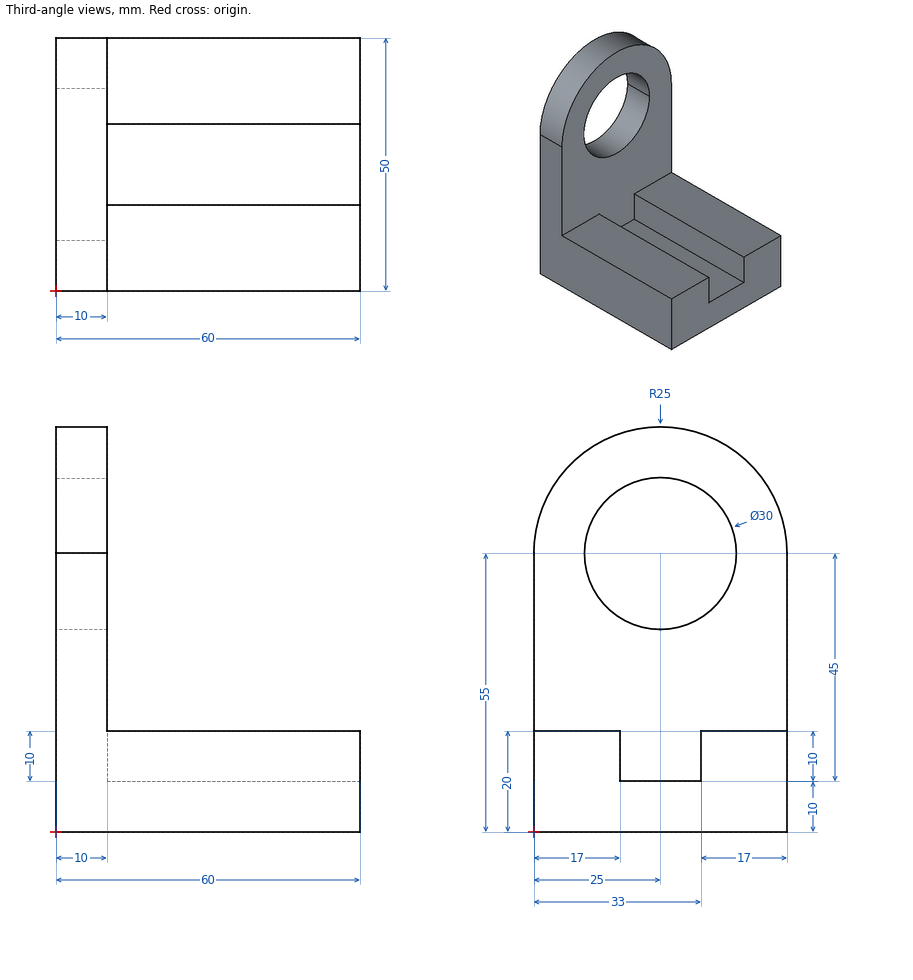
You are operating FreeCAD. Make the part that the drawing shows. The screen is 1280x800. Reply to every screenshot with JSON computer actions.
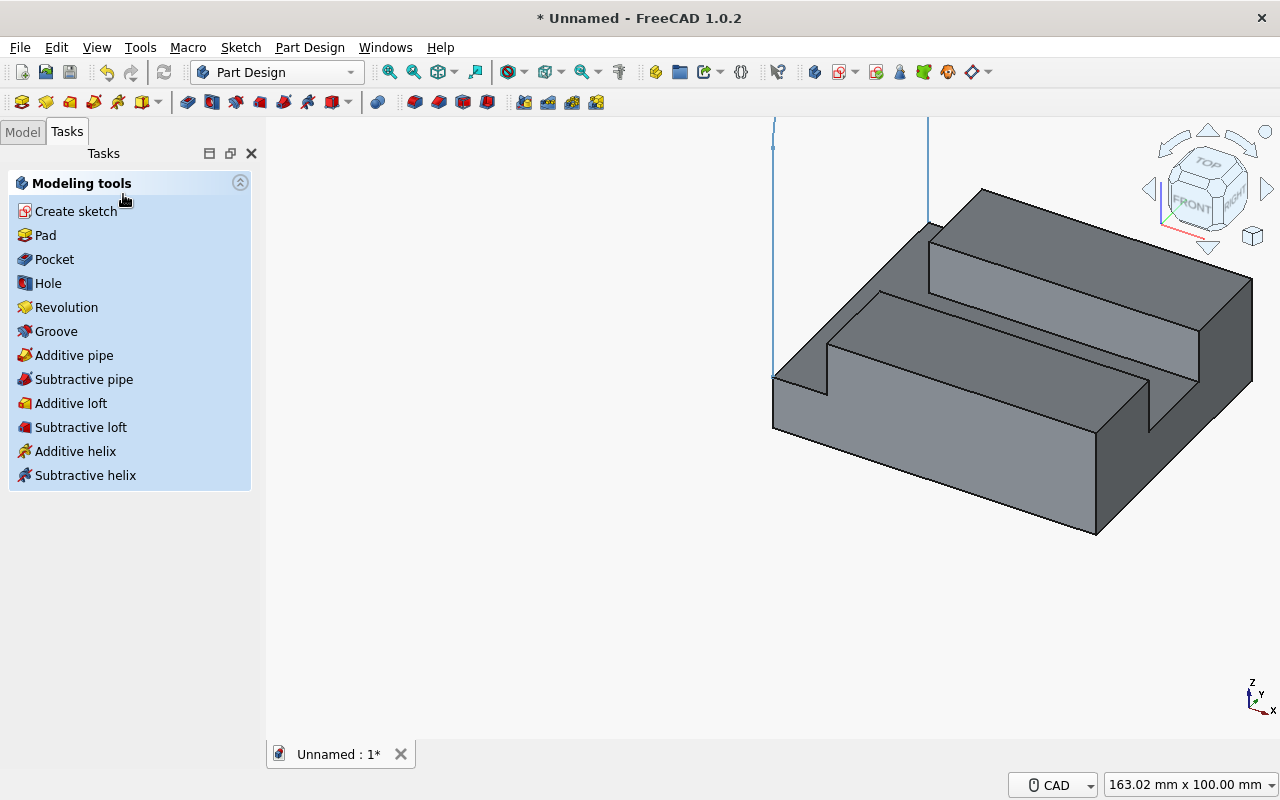
{"action": "left_click", "coordinate": [22, 102]}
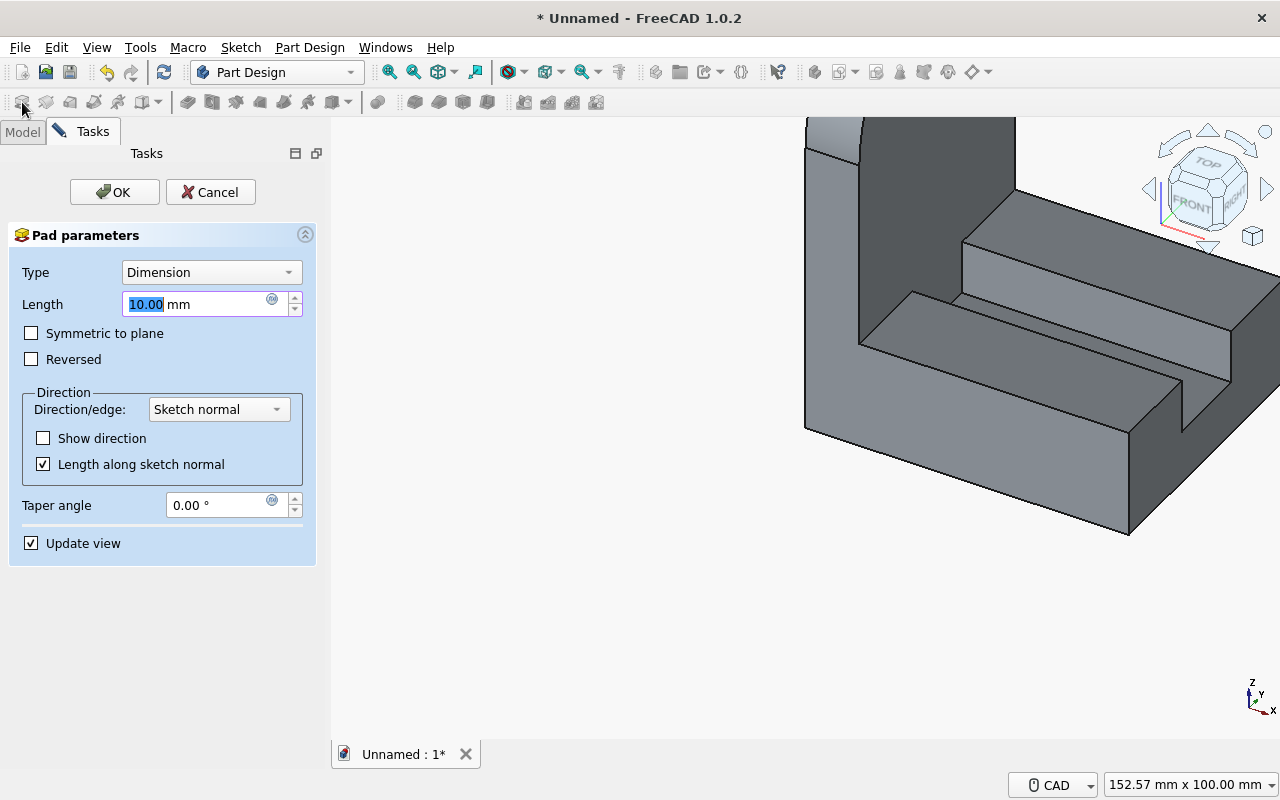
{"action": "type", "text": "10"}
{"action": "key", "text": "Tab"}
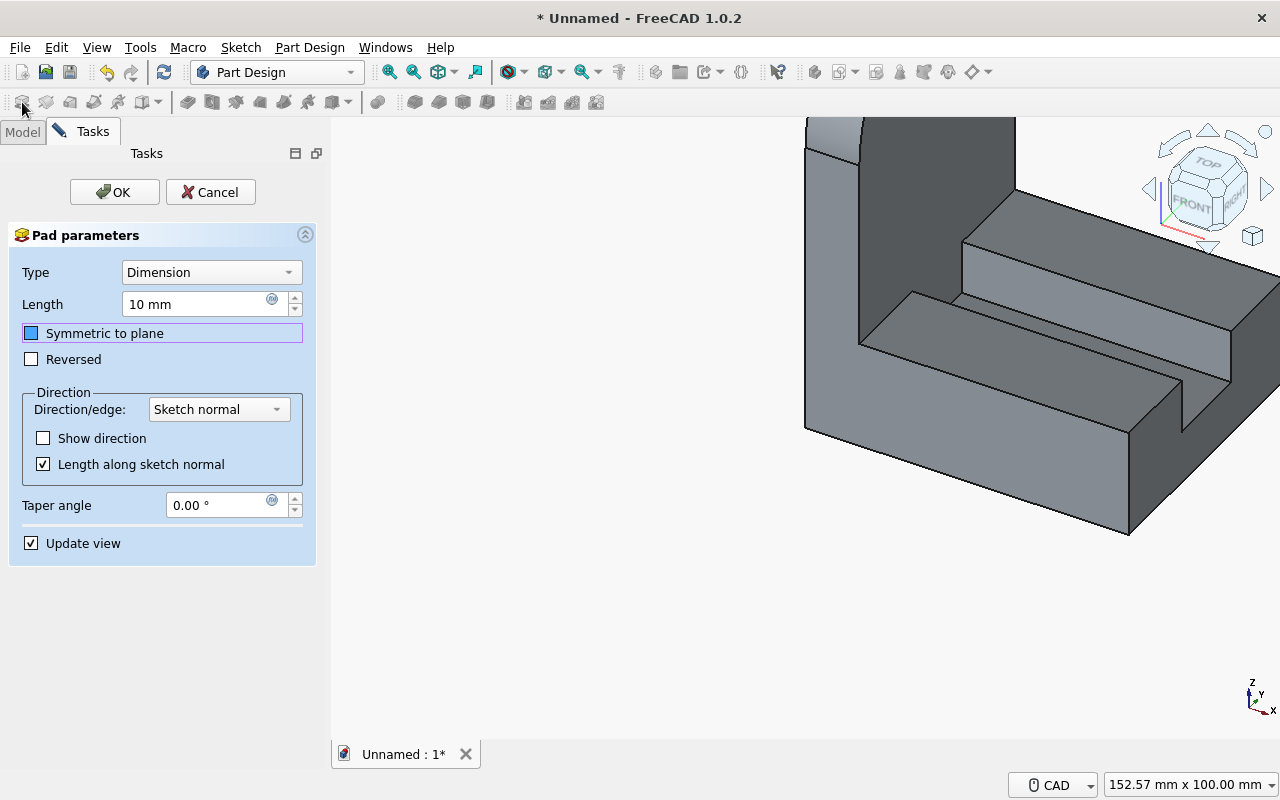
{"action": "left_click", "coordinate": [115, 192]}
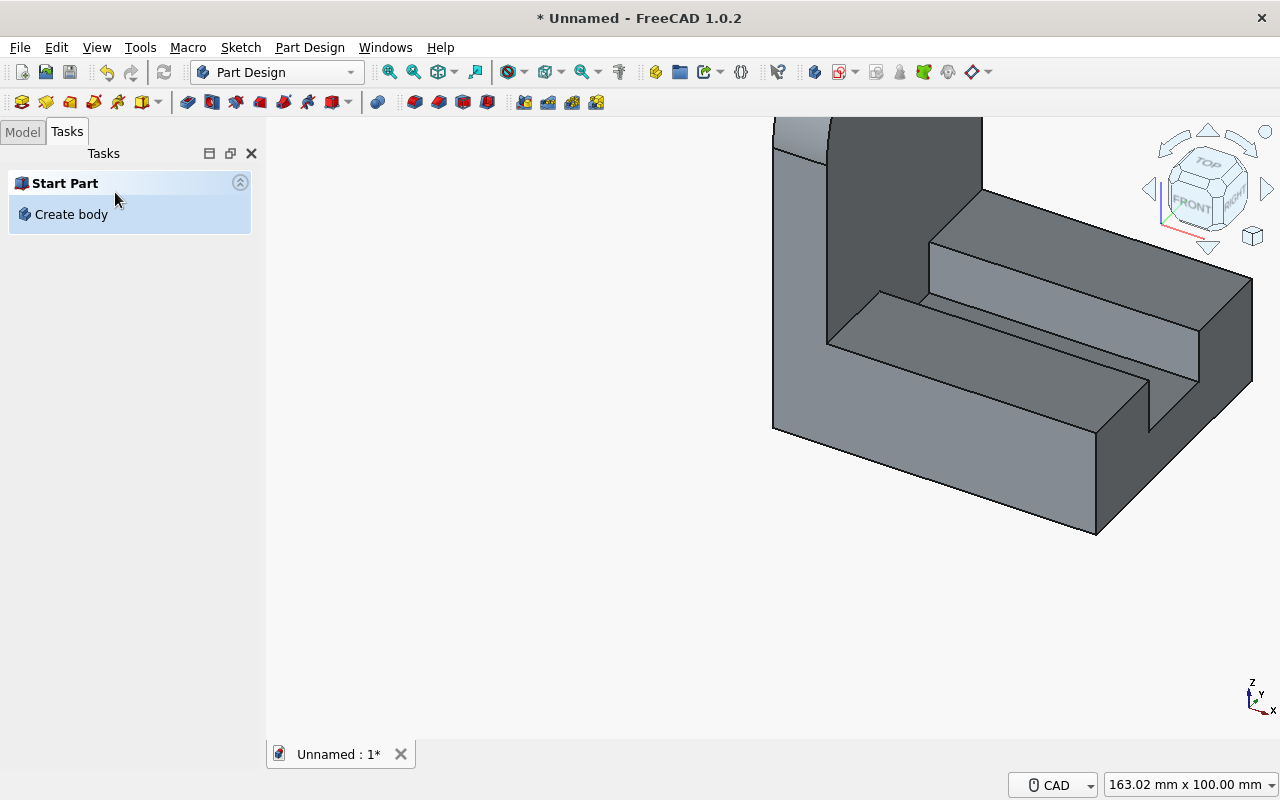
{"action": "left_click", "coordinate": [390, 72]}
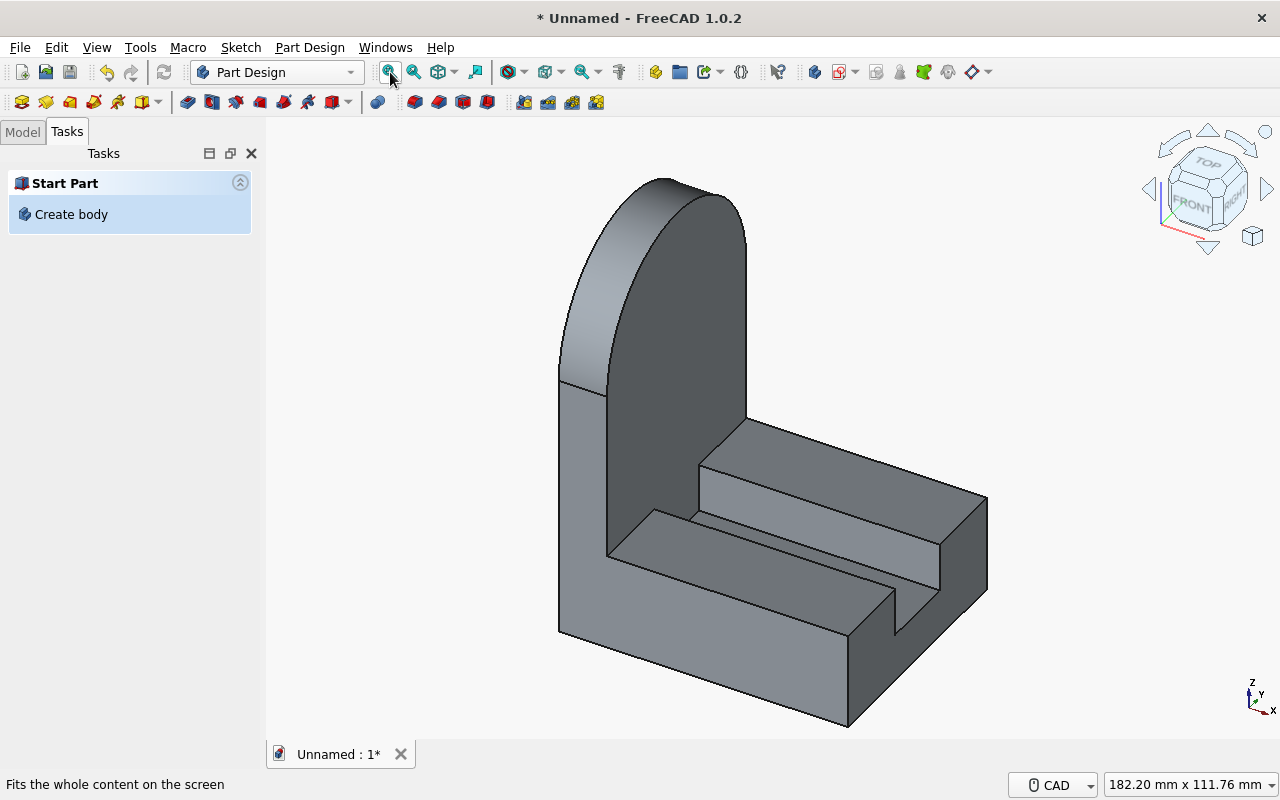
{"action": "left_click", "coordinate": [677, 327]}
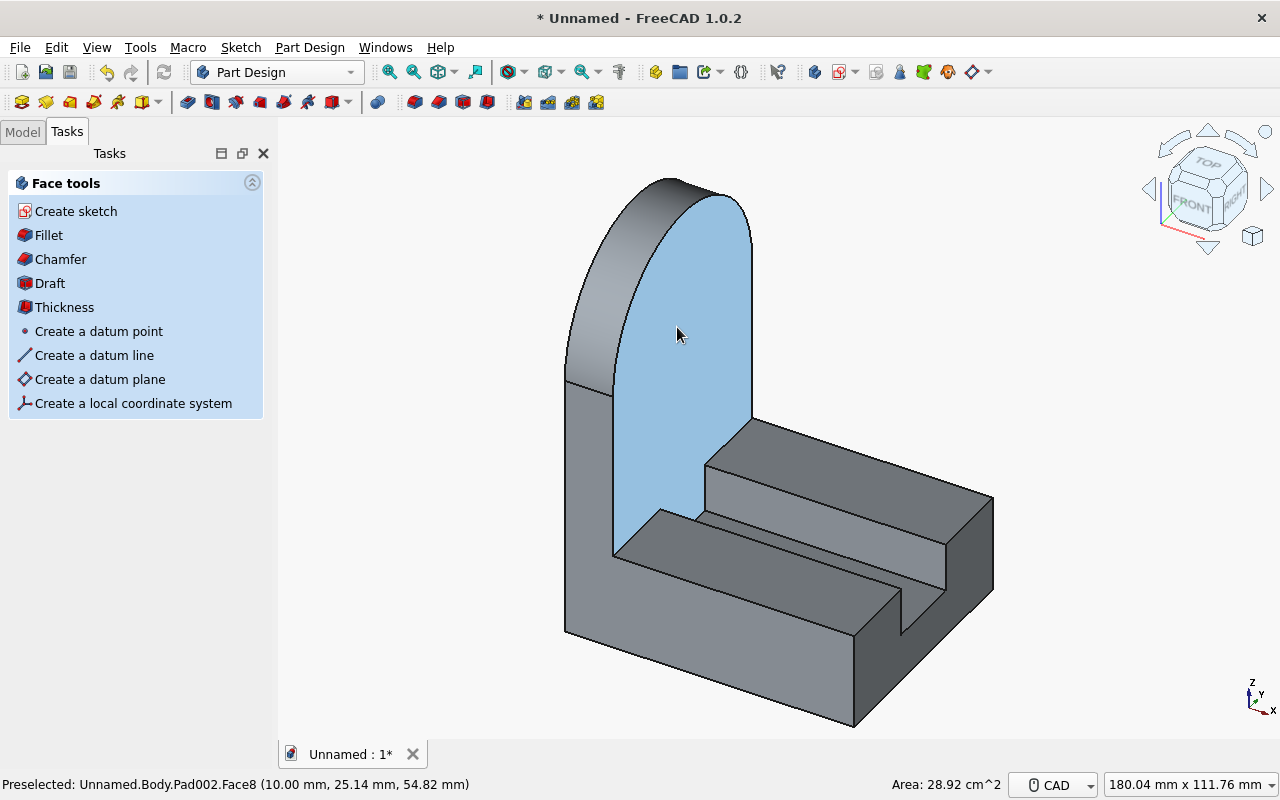
{"action": "left_click", "coordinate": [840, 72]}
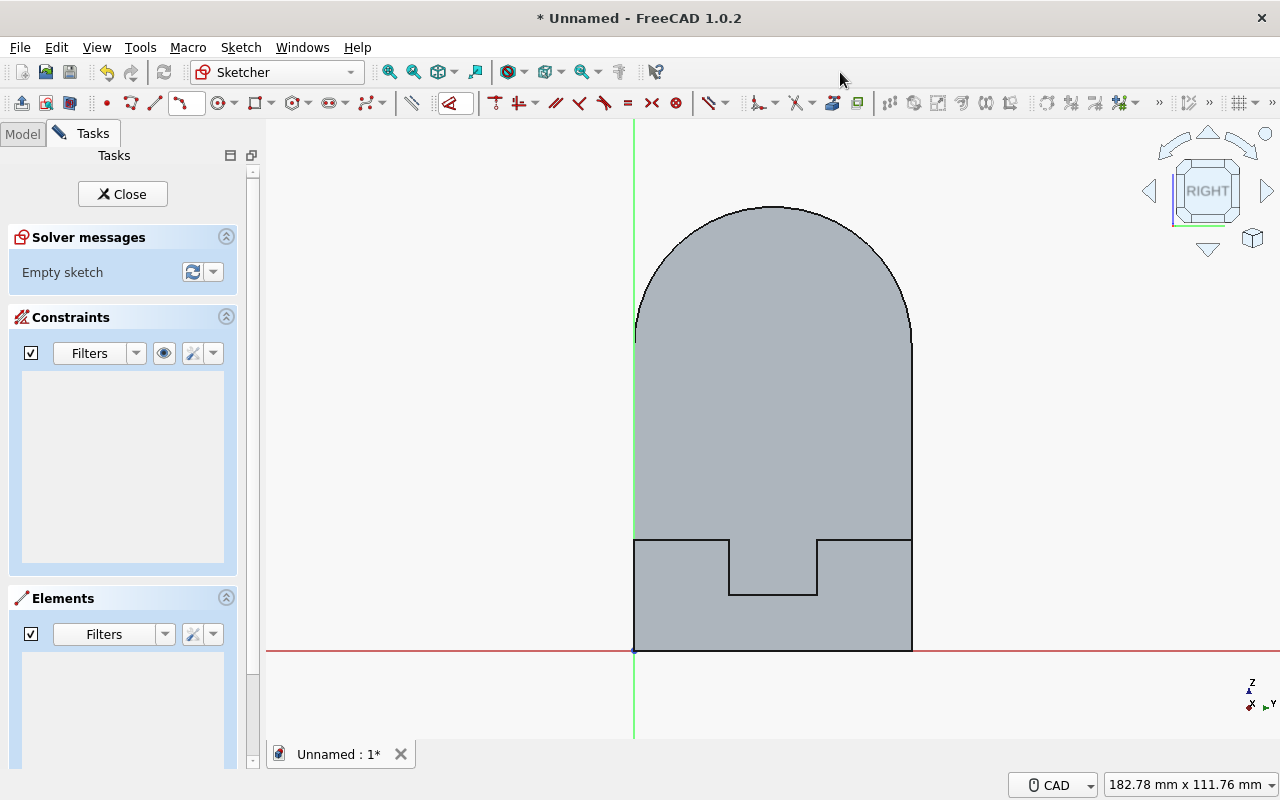
{"action": "left_click", "coordinate": [70, 104]}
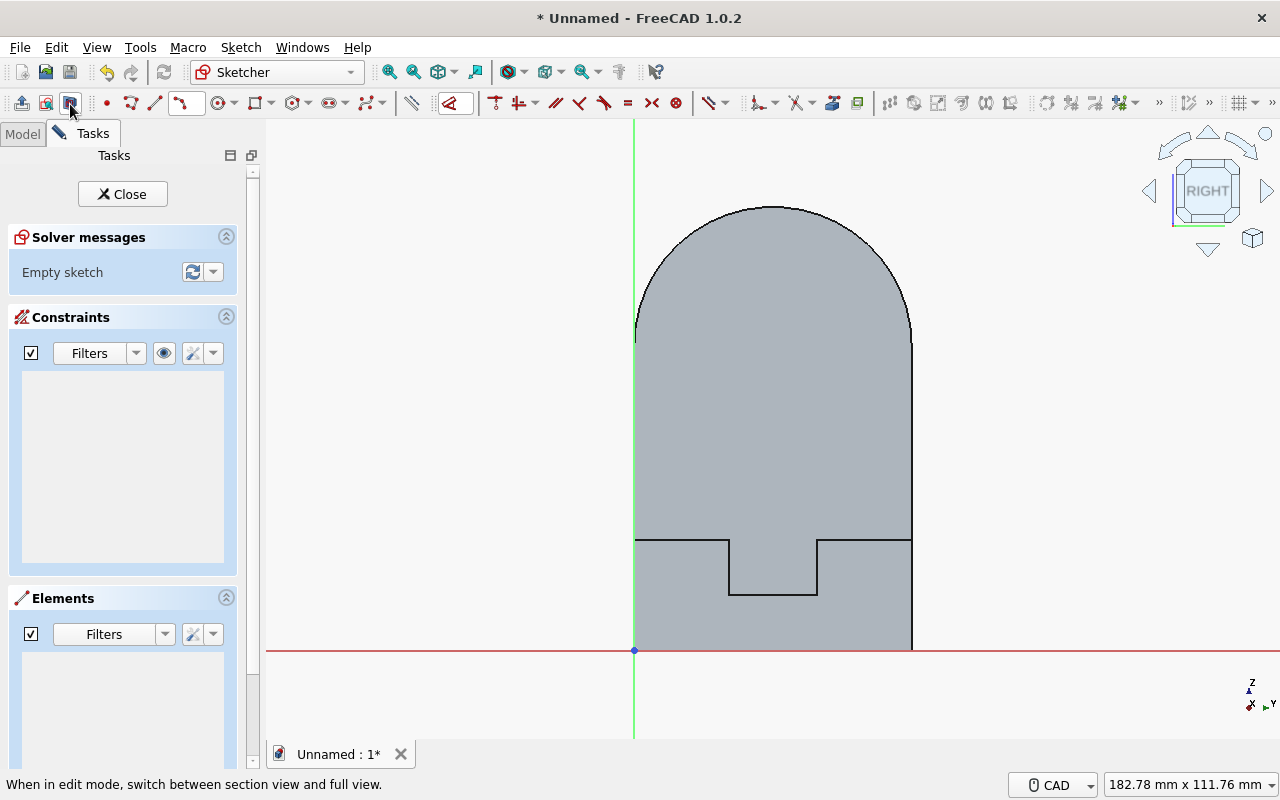
{"action": "left_click", "coordinate": [218, 104]}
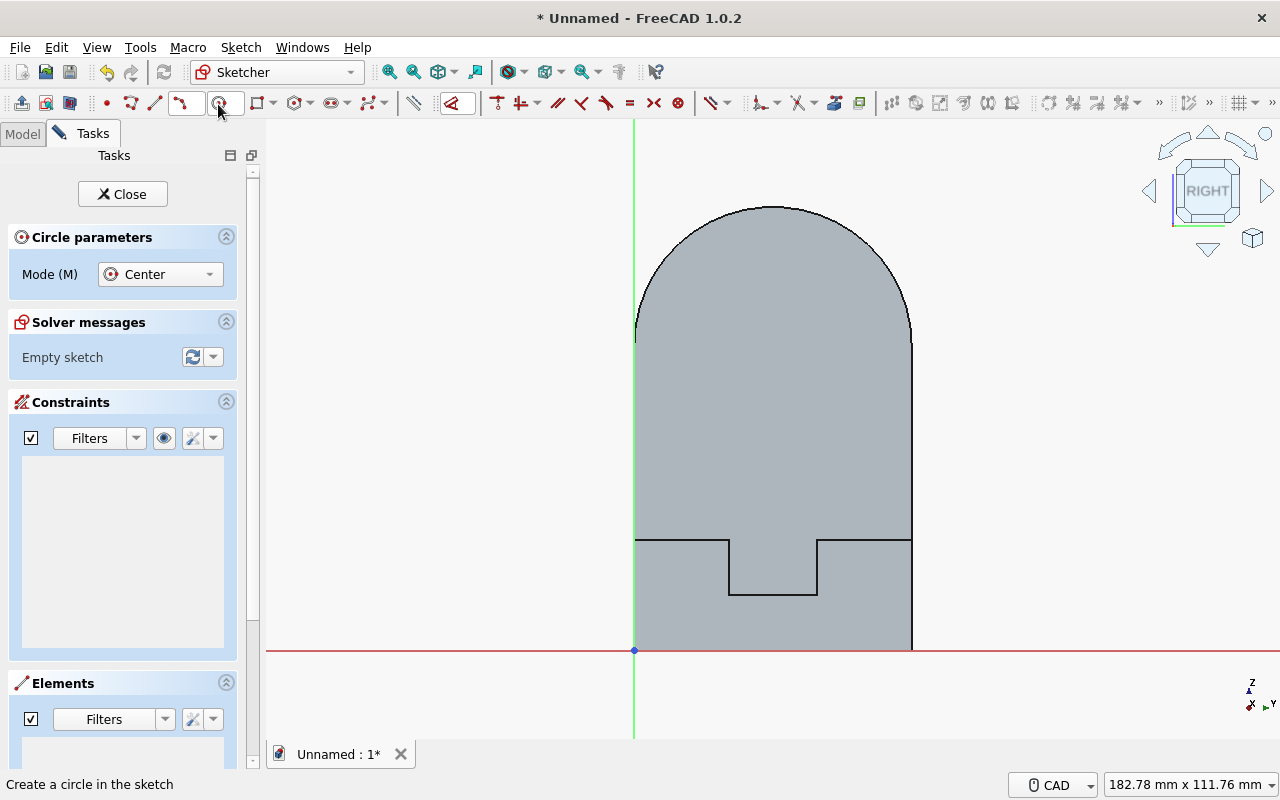
{"action": "left_click", "coordinate": [773, 346]}
{"action": "left_click", "coordinate": [832, 287]}
{"action": "key", "text": "Escape"}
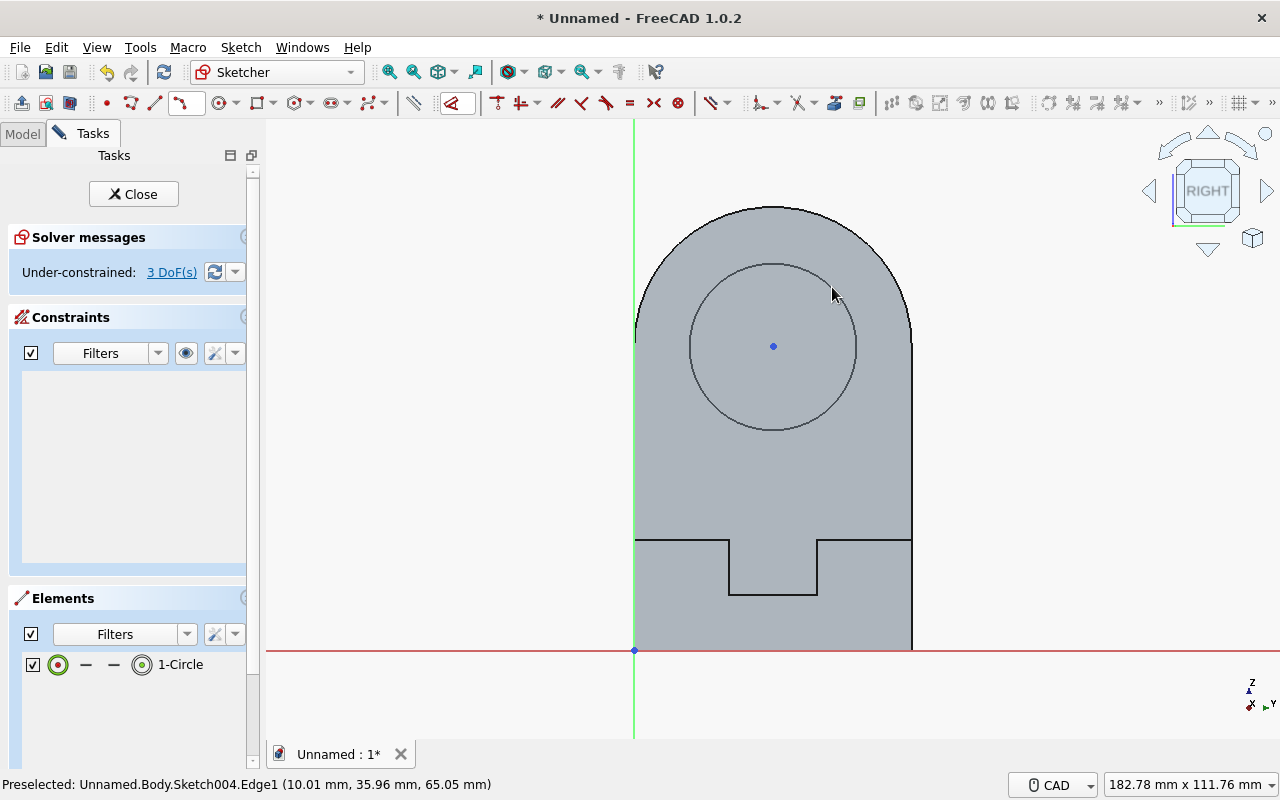
{"action": "left_click", "coordinate": [832, 288]}